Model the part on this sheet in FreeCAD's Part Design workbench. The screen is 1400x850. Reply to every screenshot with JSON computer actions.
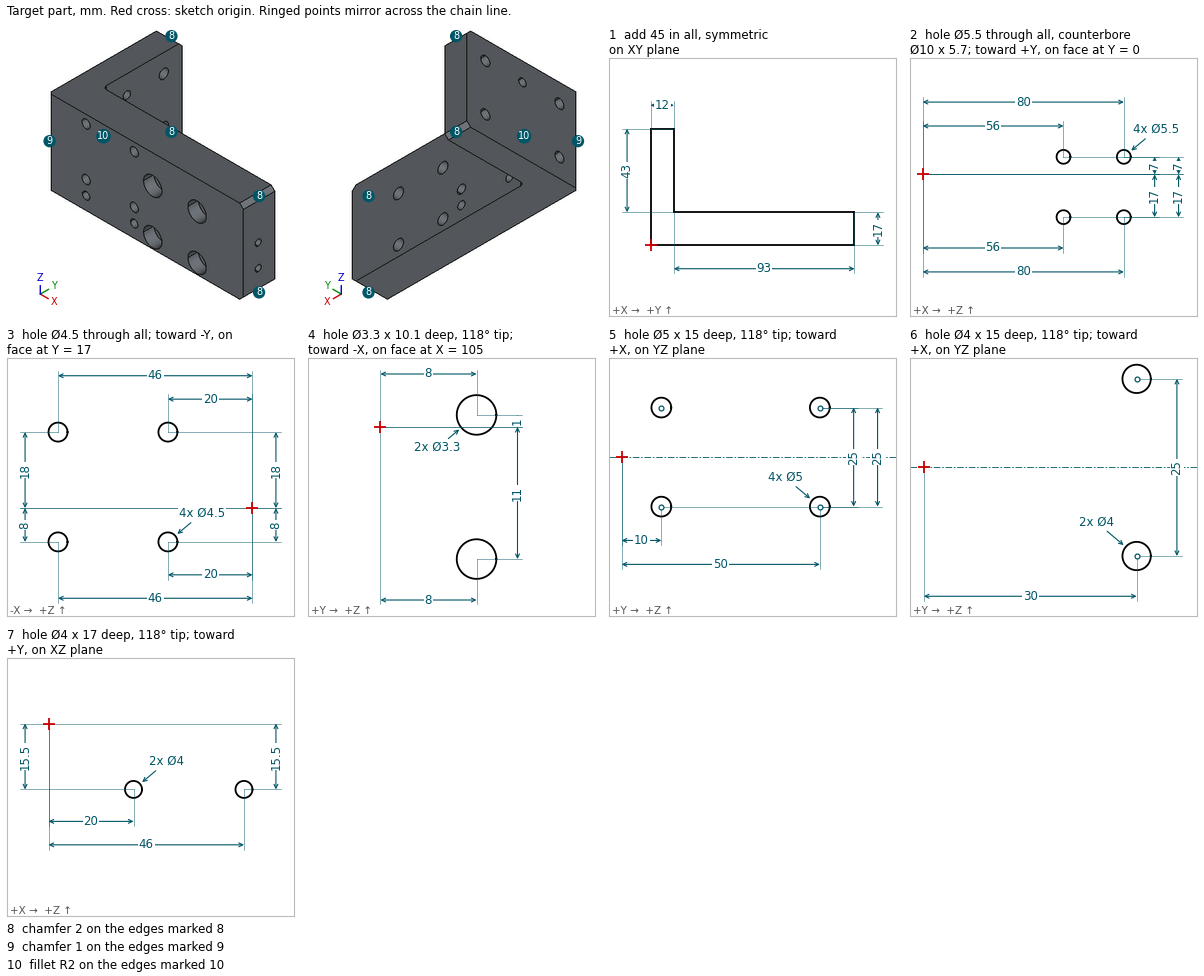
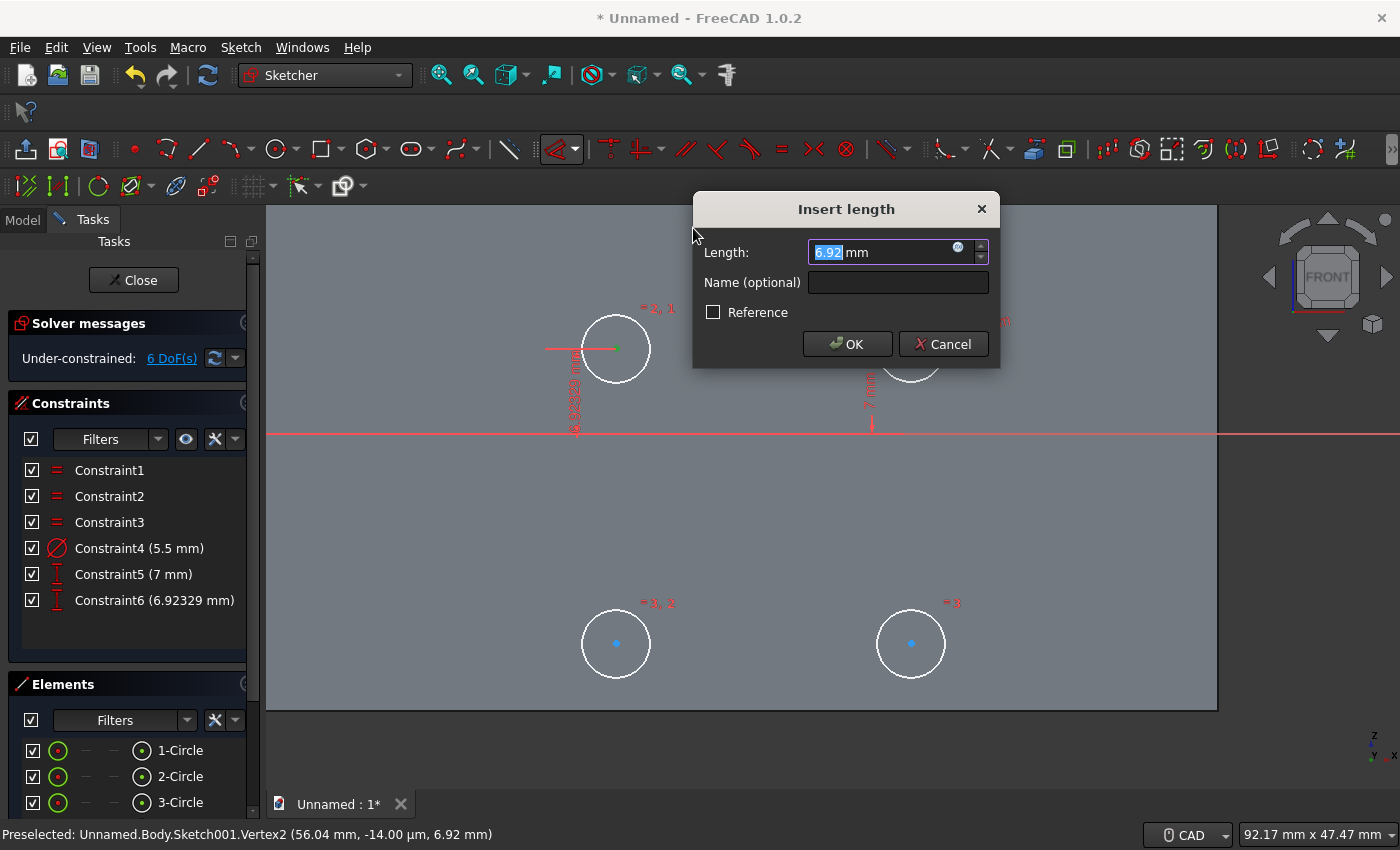
{"action": "type", "text": "7"}
{"action": "key", "text": "Return"}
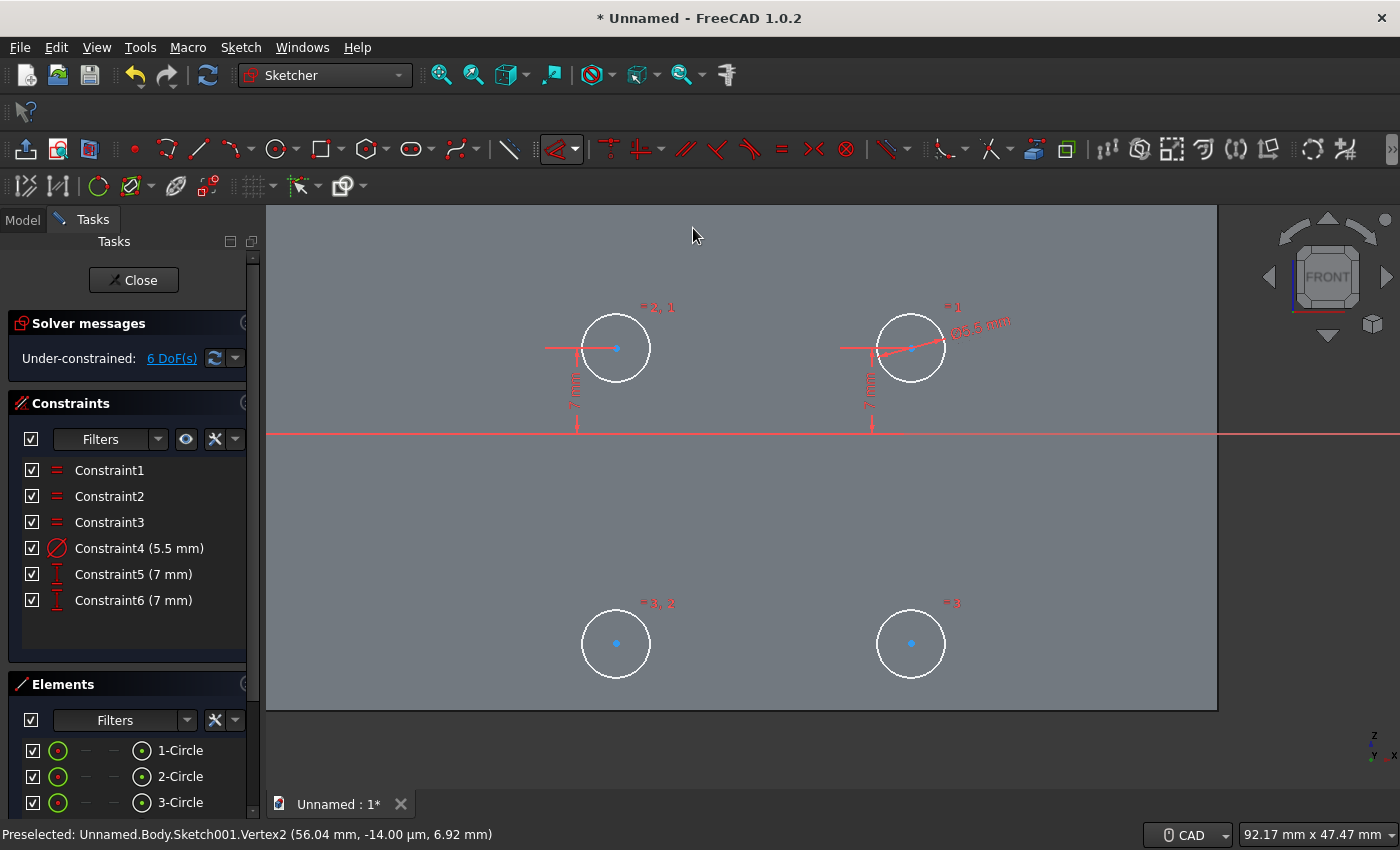
{"action": "left_click", "coordinate": [911, 348]}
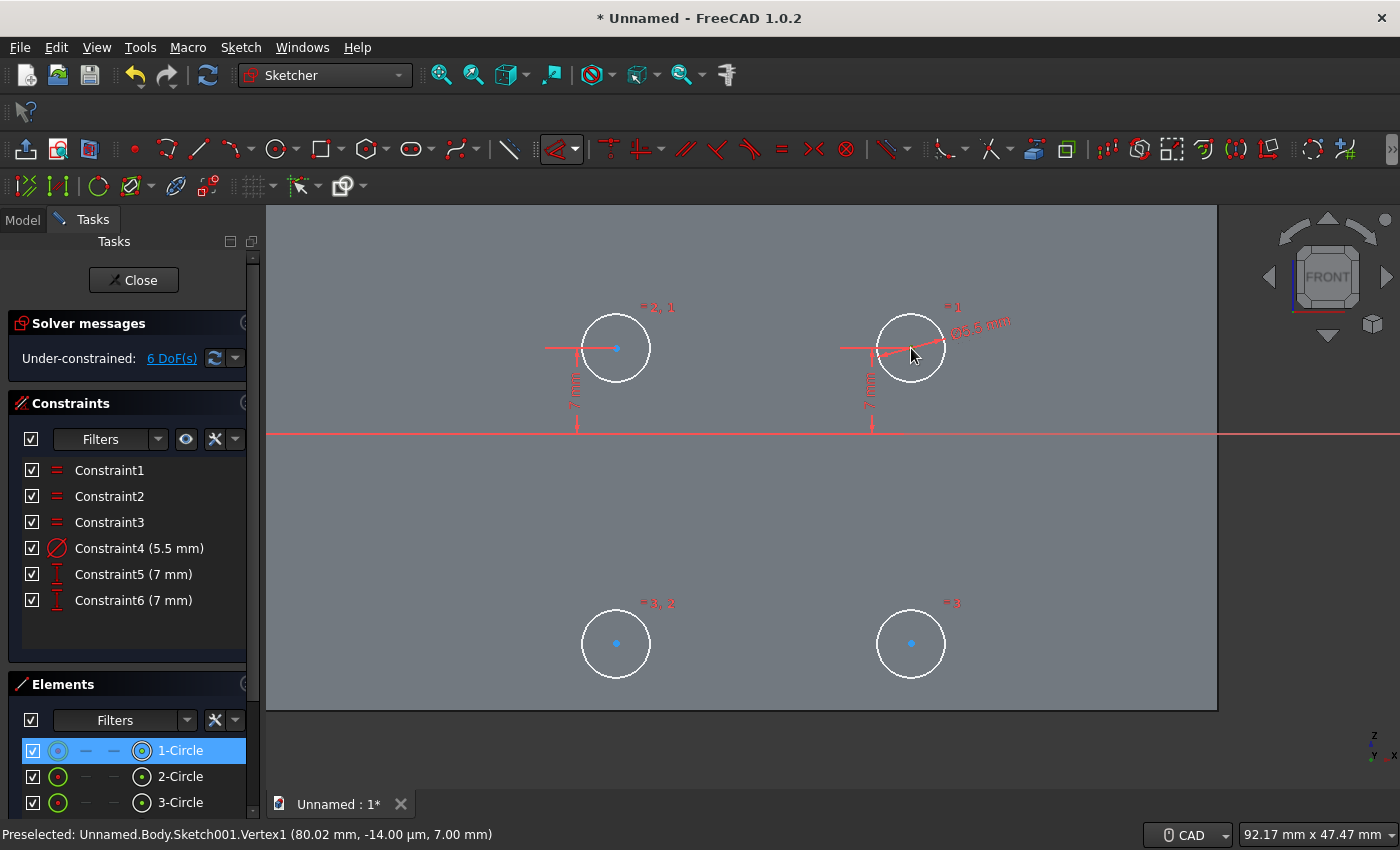
{"action": "key", "text": "l"}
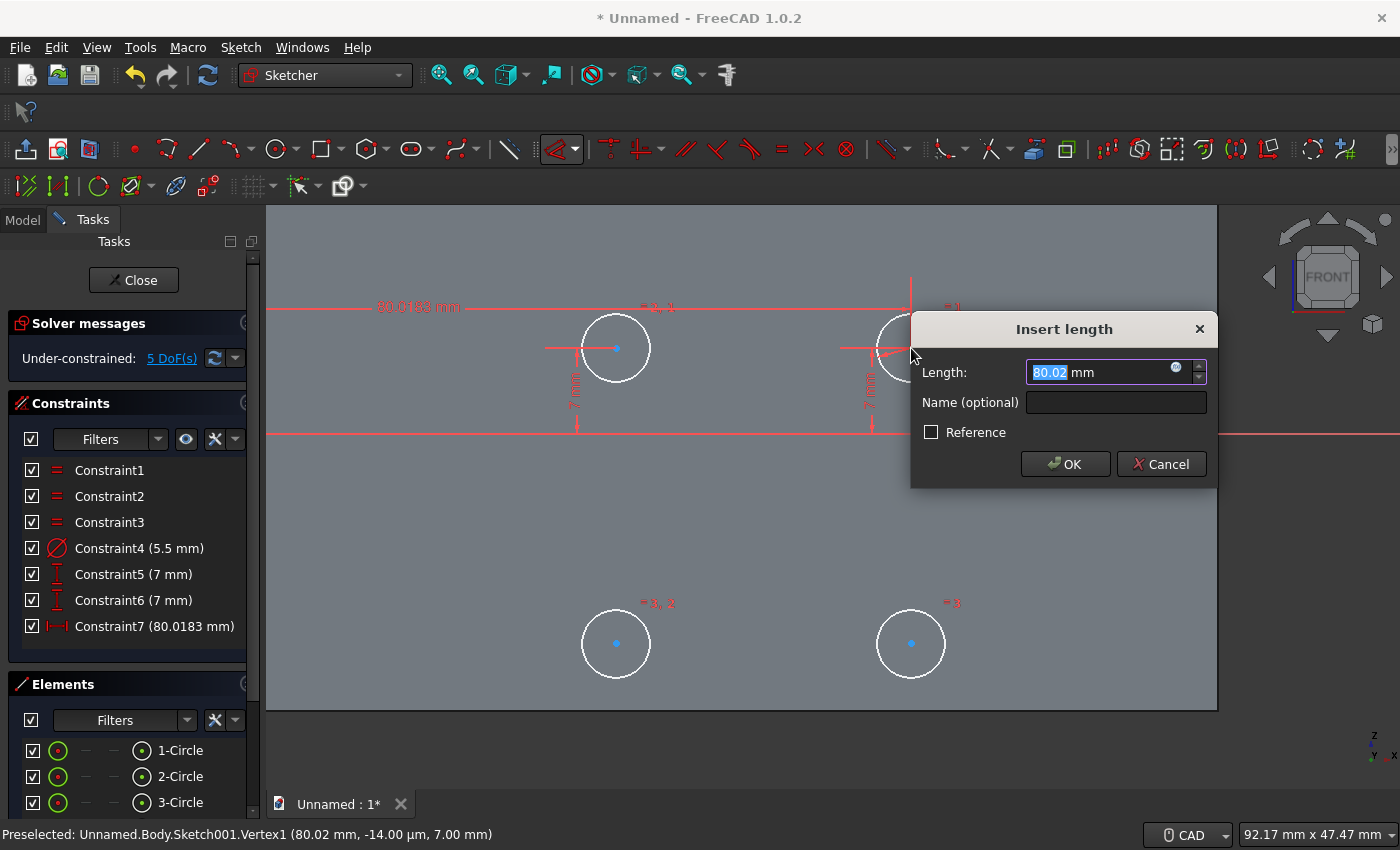
{"action": "type", "text": "80"}
{"action": "key", "text": "Return"}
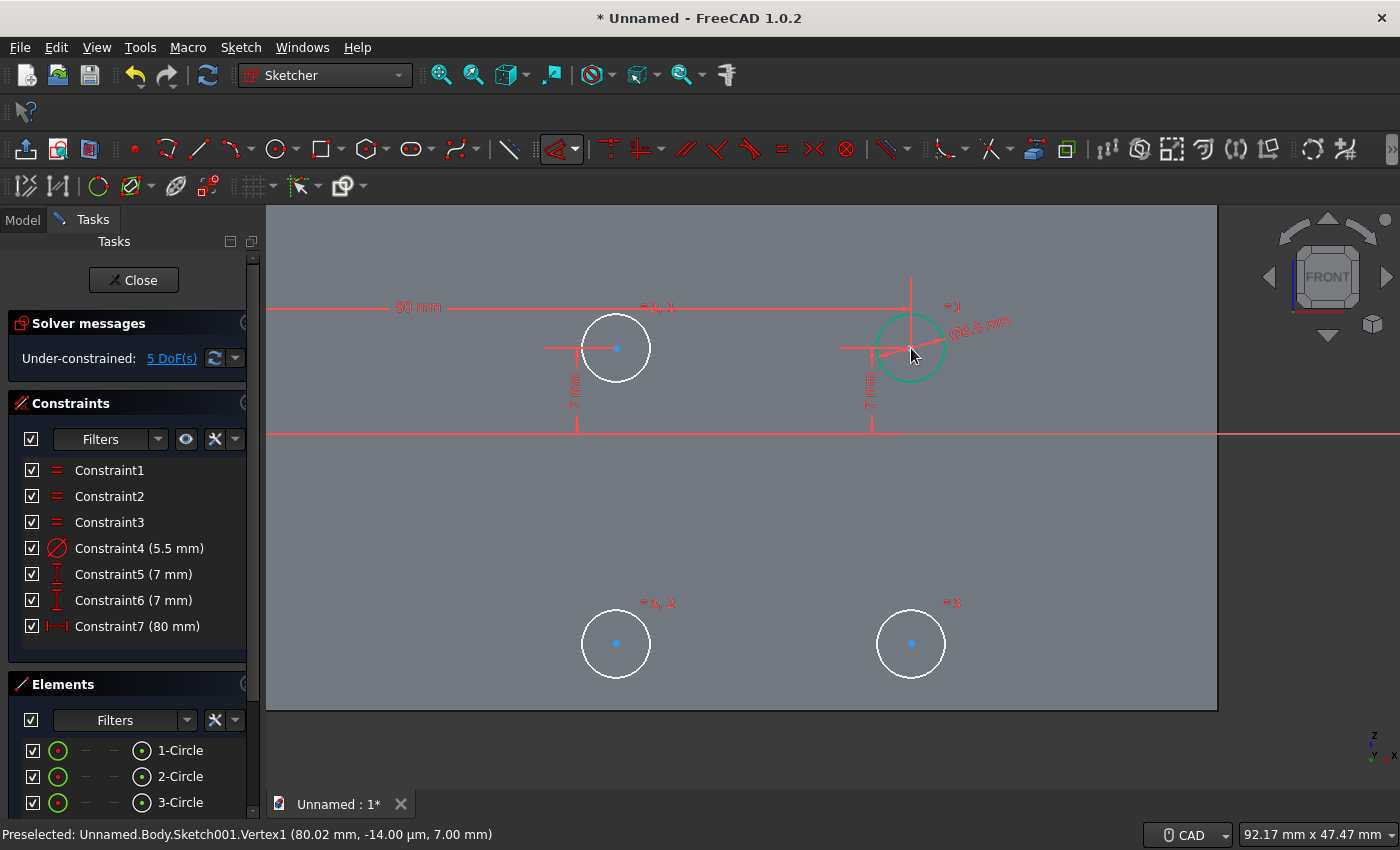
{"action": "left_click", "coordinate": [616, 348]}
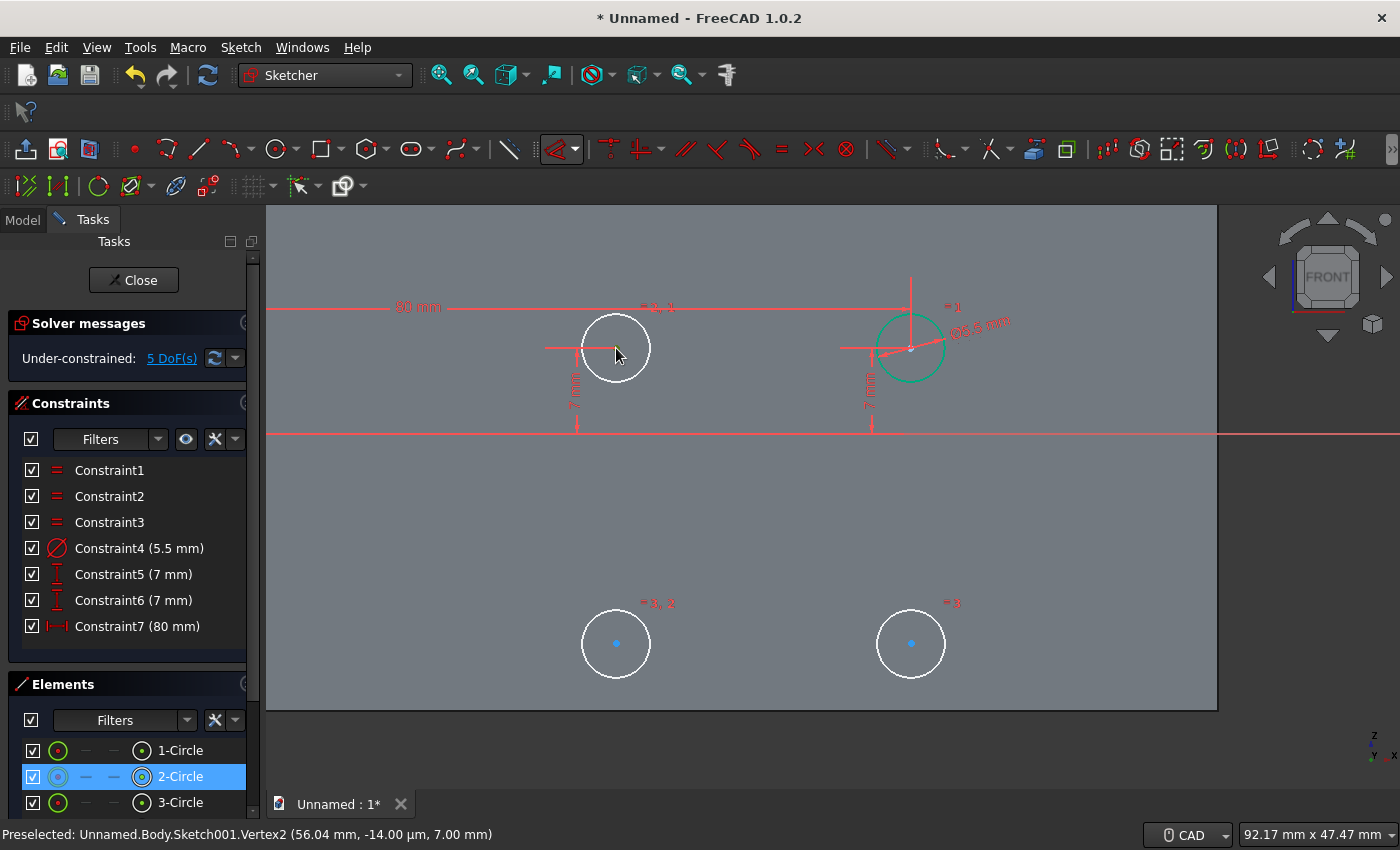
{"action": "key", "text": "l"}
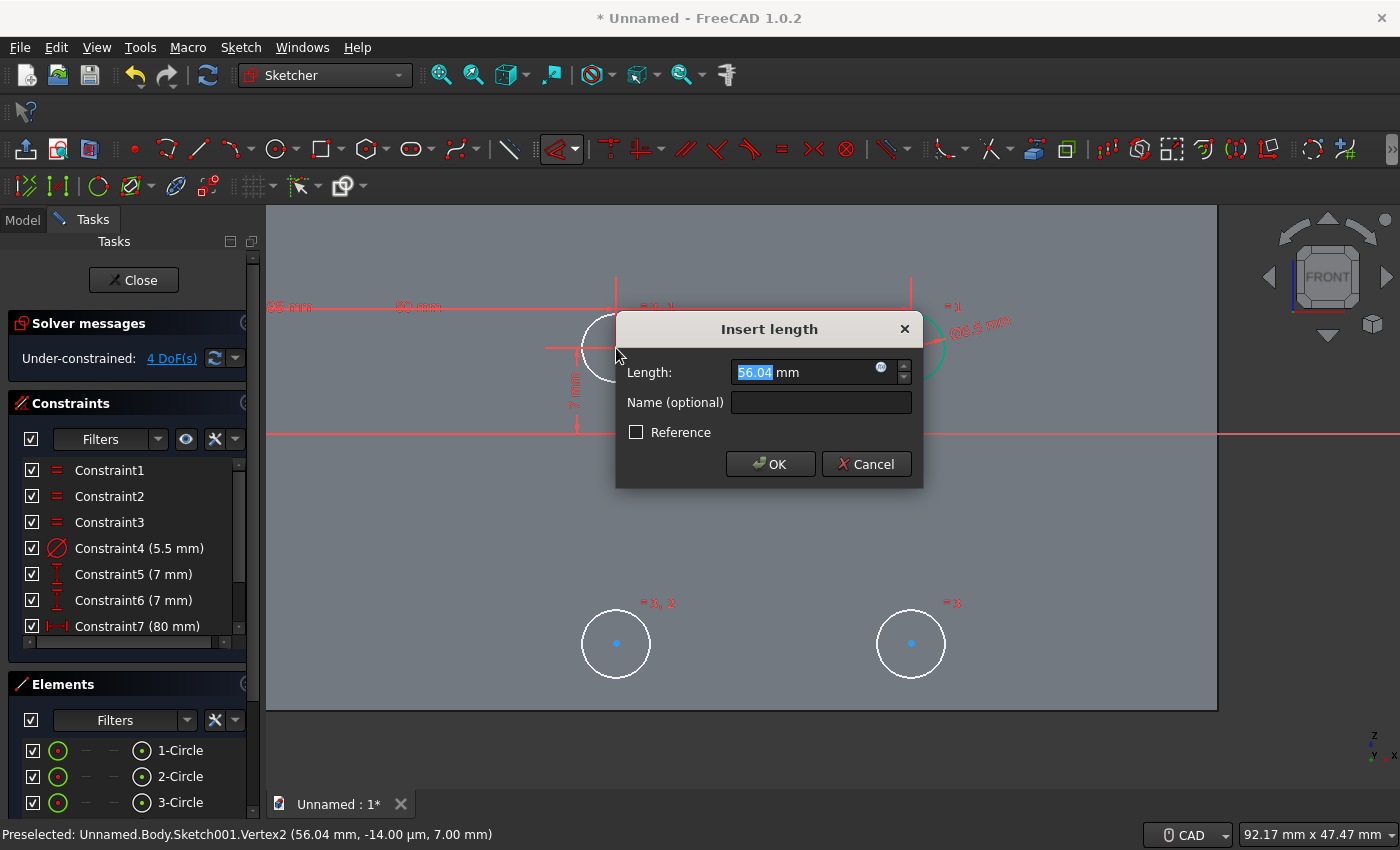
{"action": "type", "text": "56"}
{"action": "key", "text": "Return"}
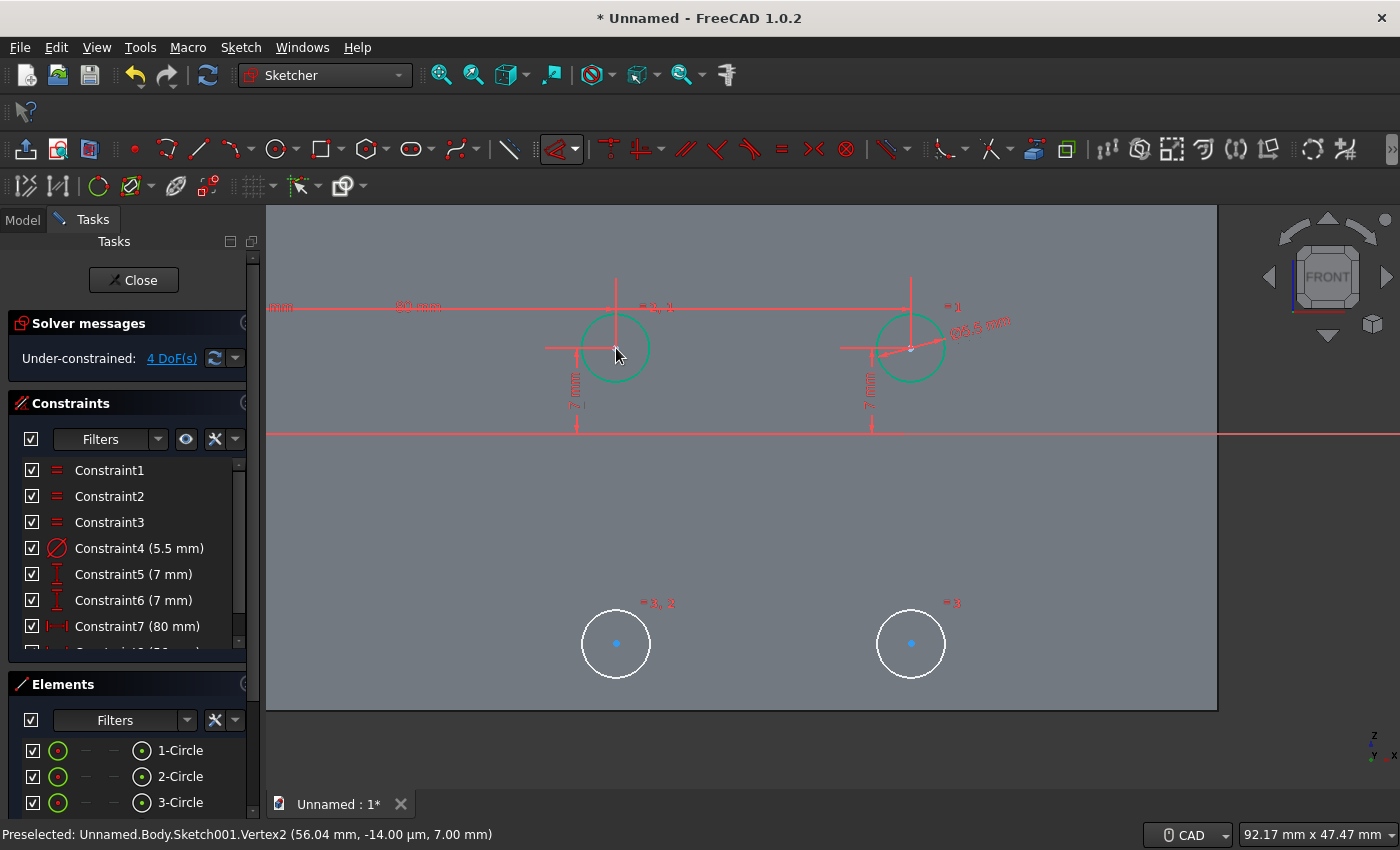
{"action": "left_click", "coordinate": [616, 644]}